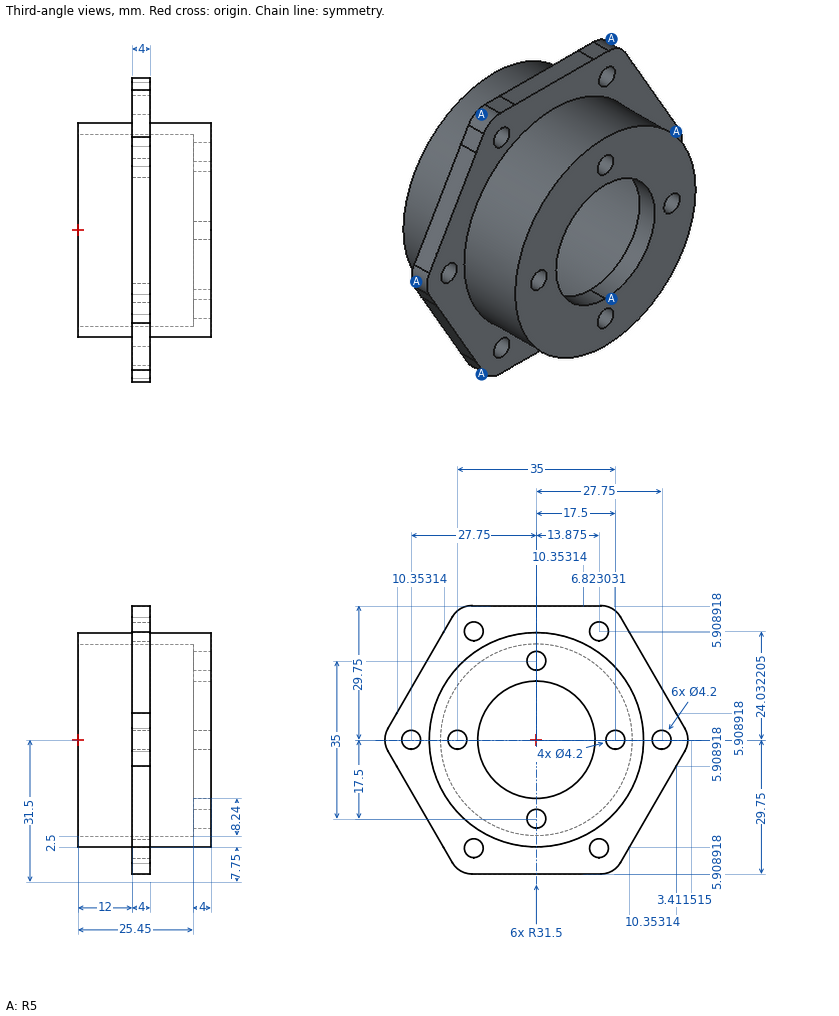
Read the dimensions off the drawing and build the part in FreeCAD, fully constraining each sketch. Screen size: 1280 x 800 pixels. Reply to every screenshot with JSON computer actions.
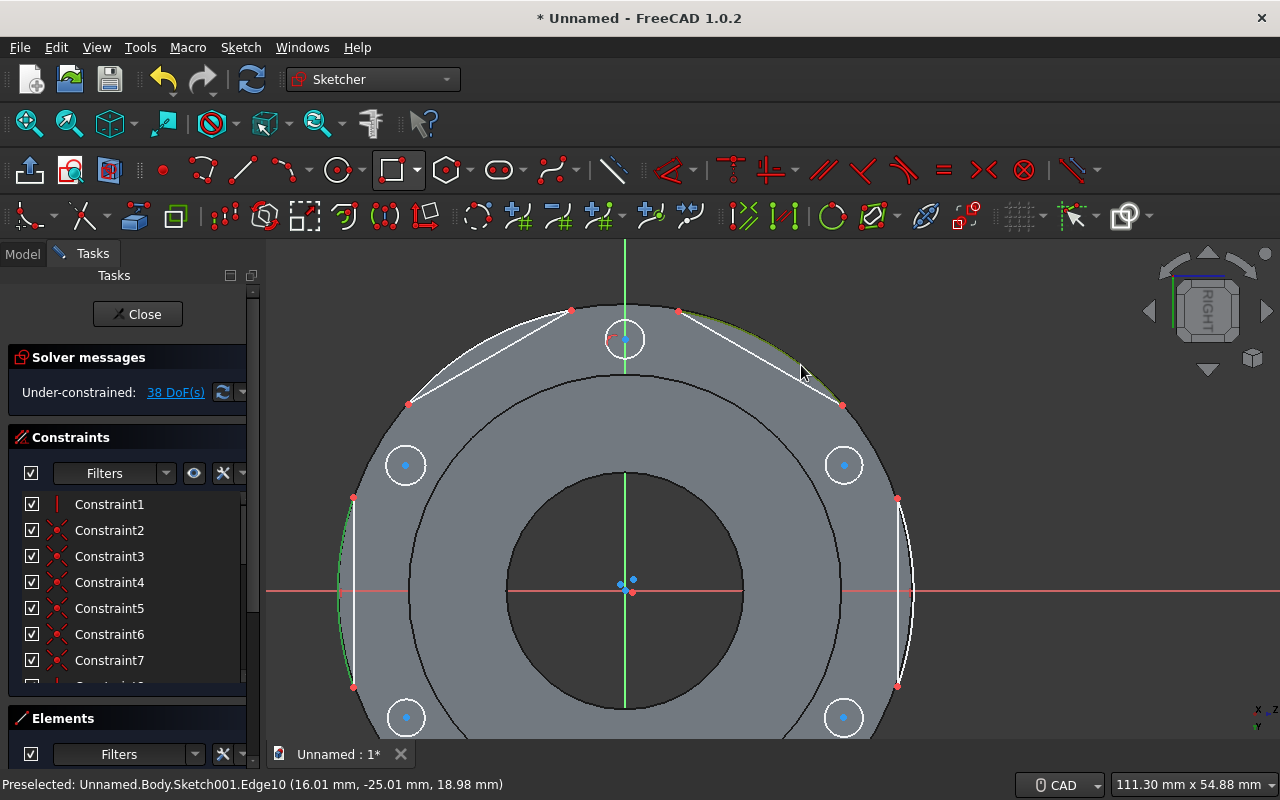
{"action": "key", "text": "c"}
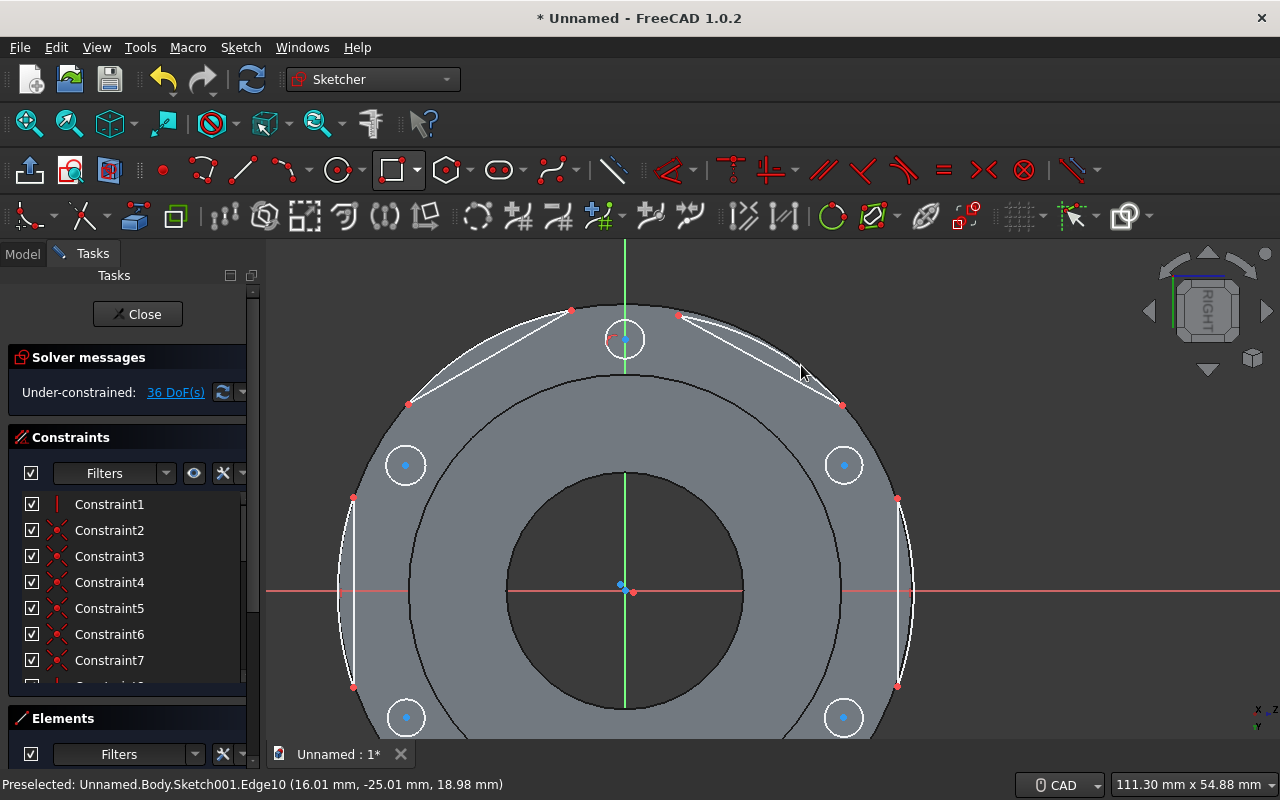
{"action": "left_click", "coordinate": [340, 554]}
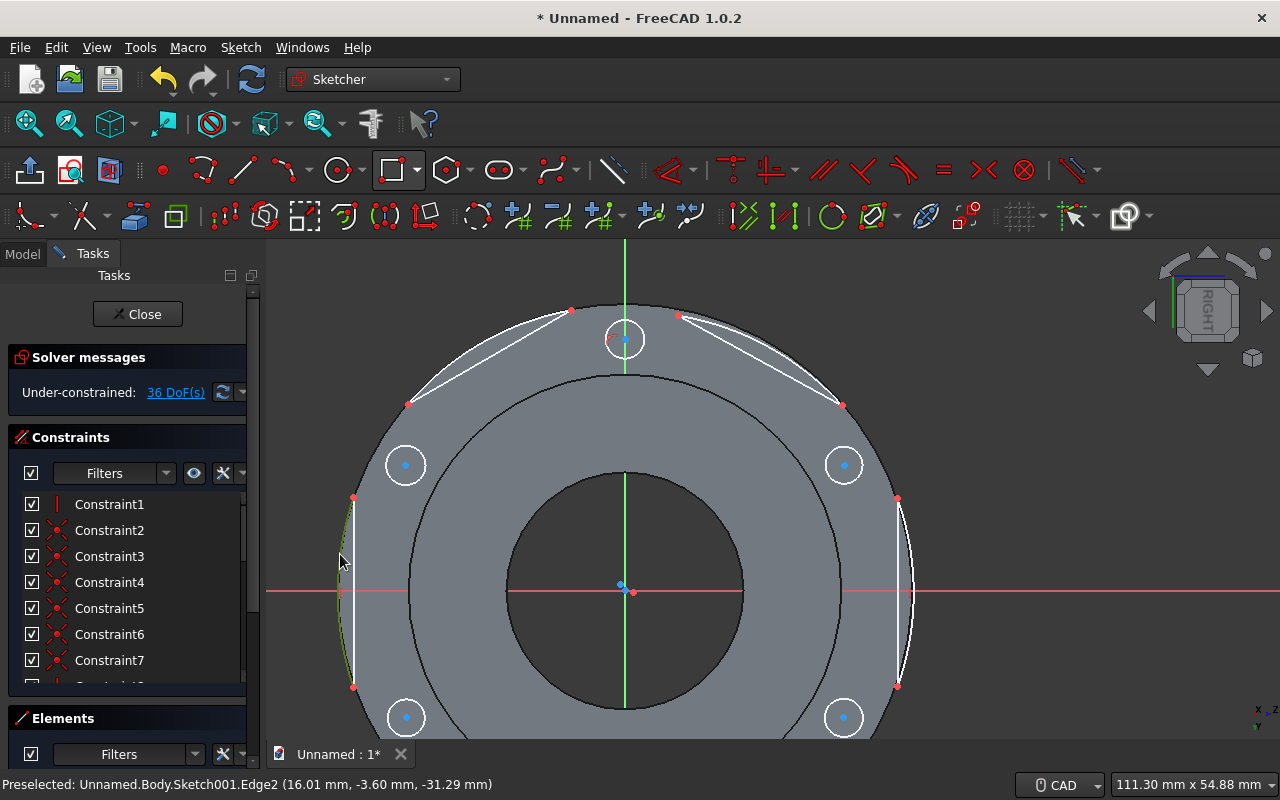
{"action": "left_click", "coordinate": [516, 326]}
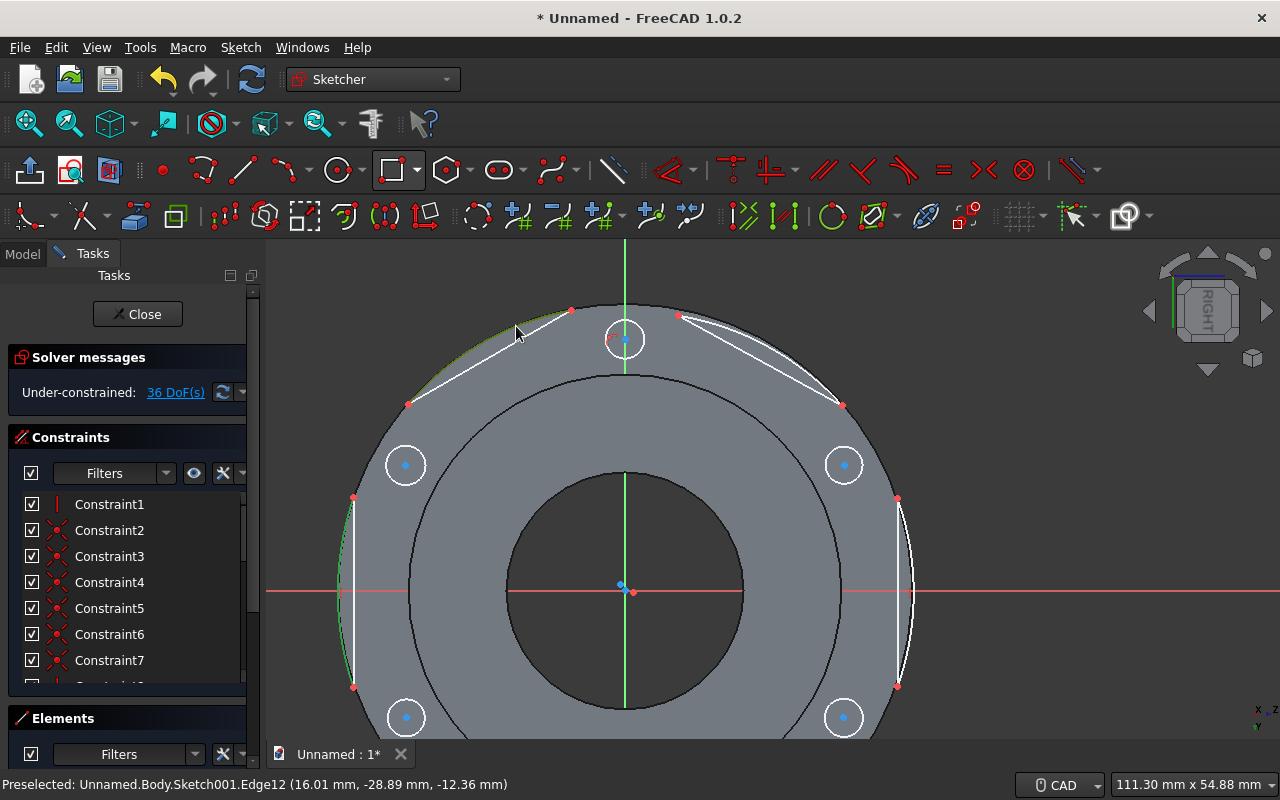
{"action": "key", "text": "c"}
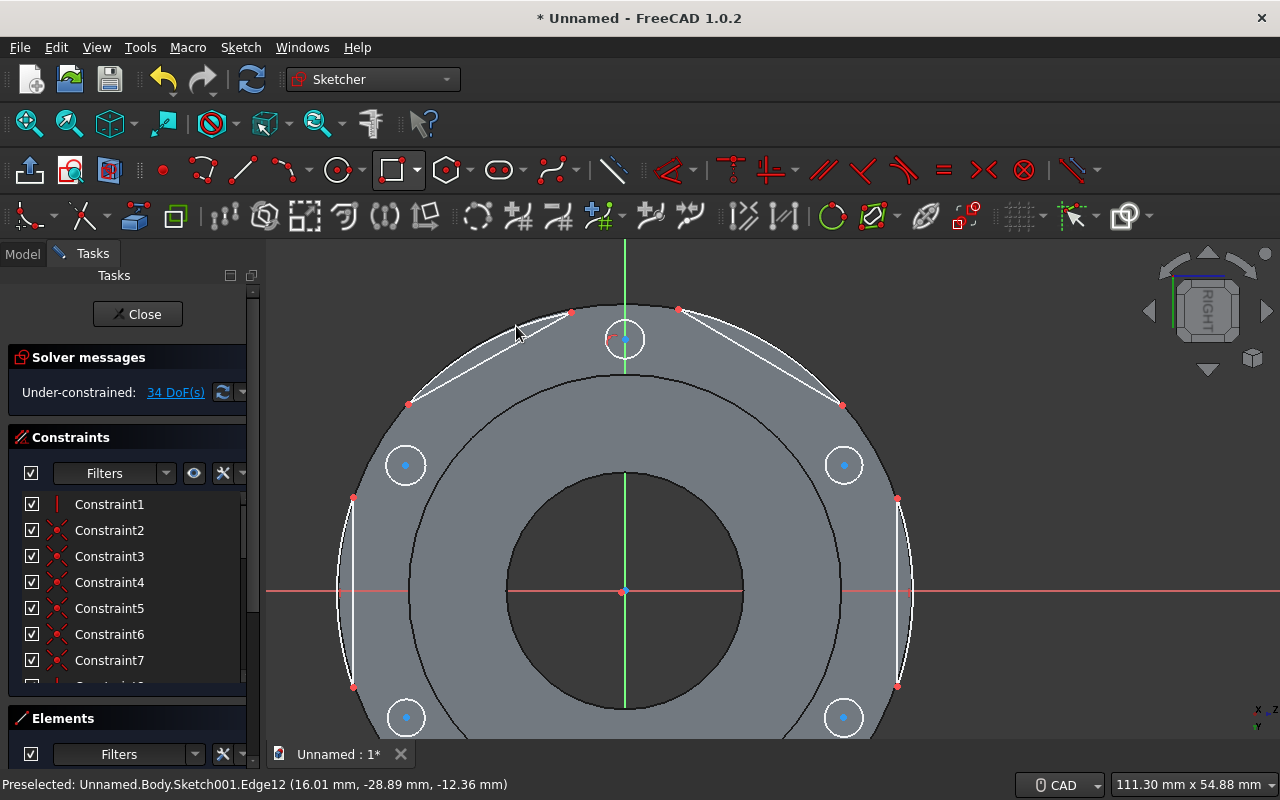
{"action": "scroll", "coordinate": [623, 592], "scroll_direction": "up", "scroll_amount": 4}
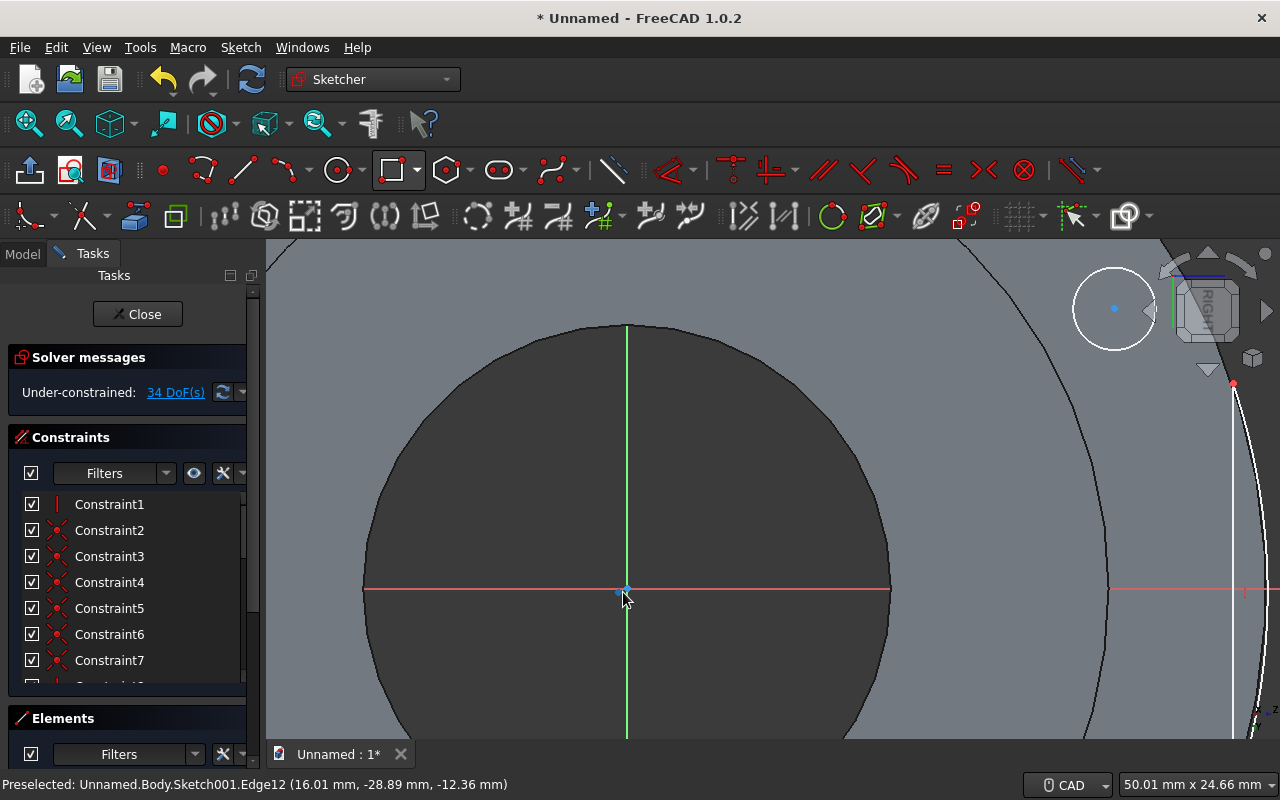
{"action": "left_click_drag", "start_coordinate": [609, 579], "coordinate": [637, 603]}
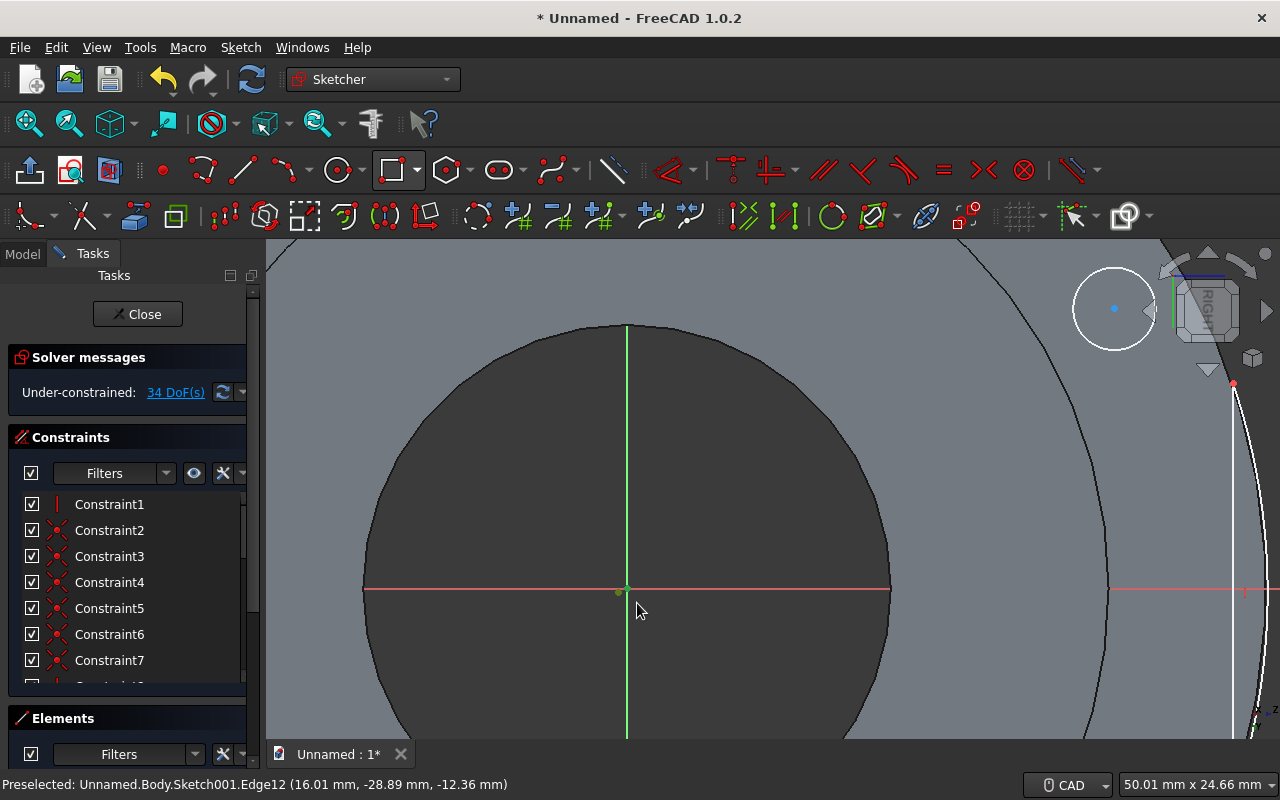
{"action": "key", "text": "c"}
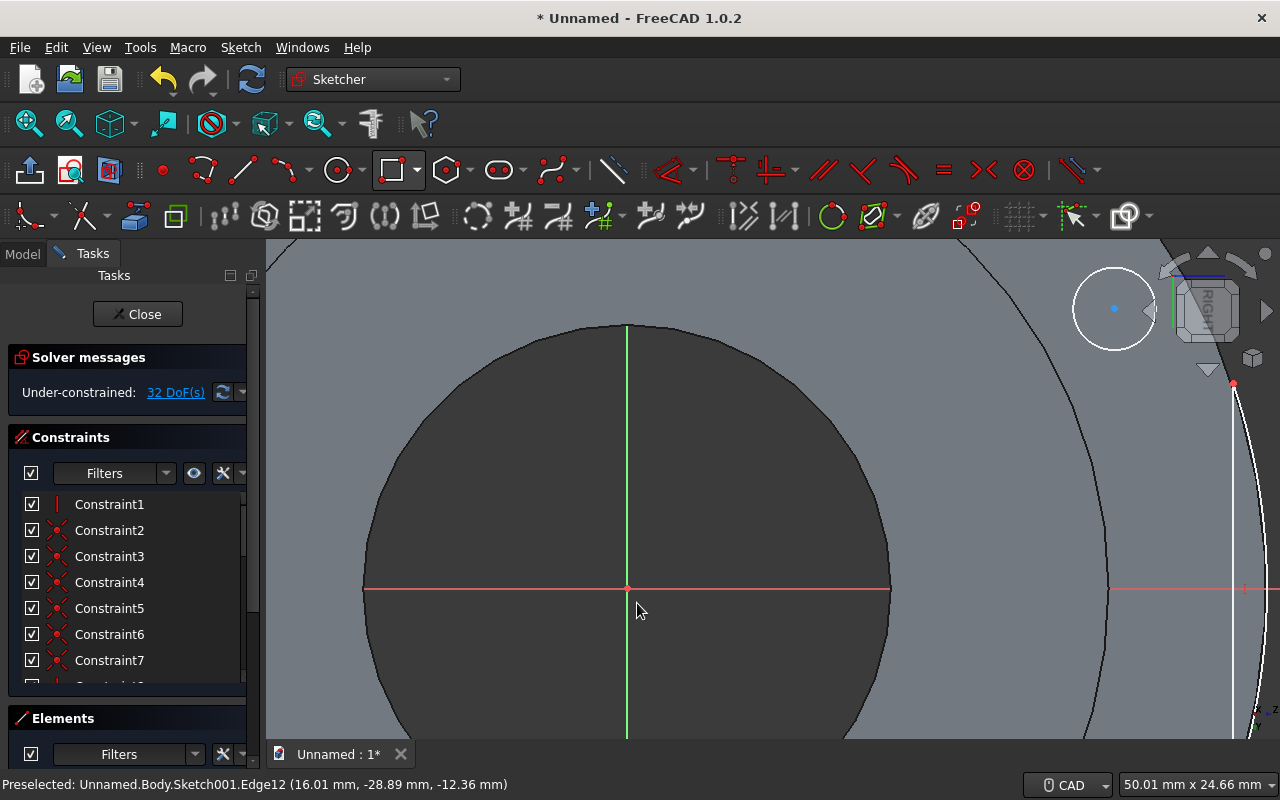
{"action": "scroll", "coordinate": [730, 456], "scroll_direction": "down", "scroll_amount": 7}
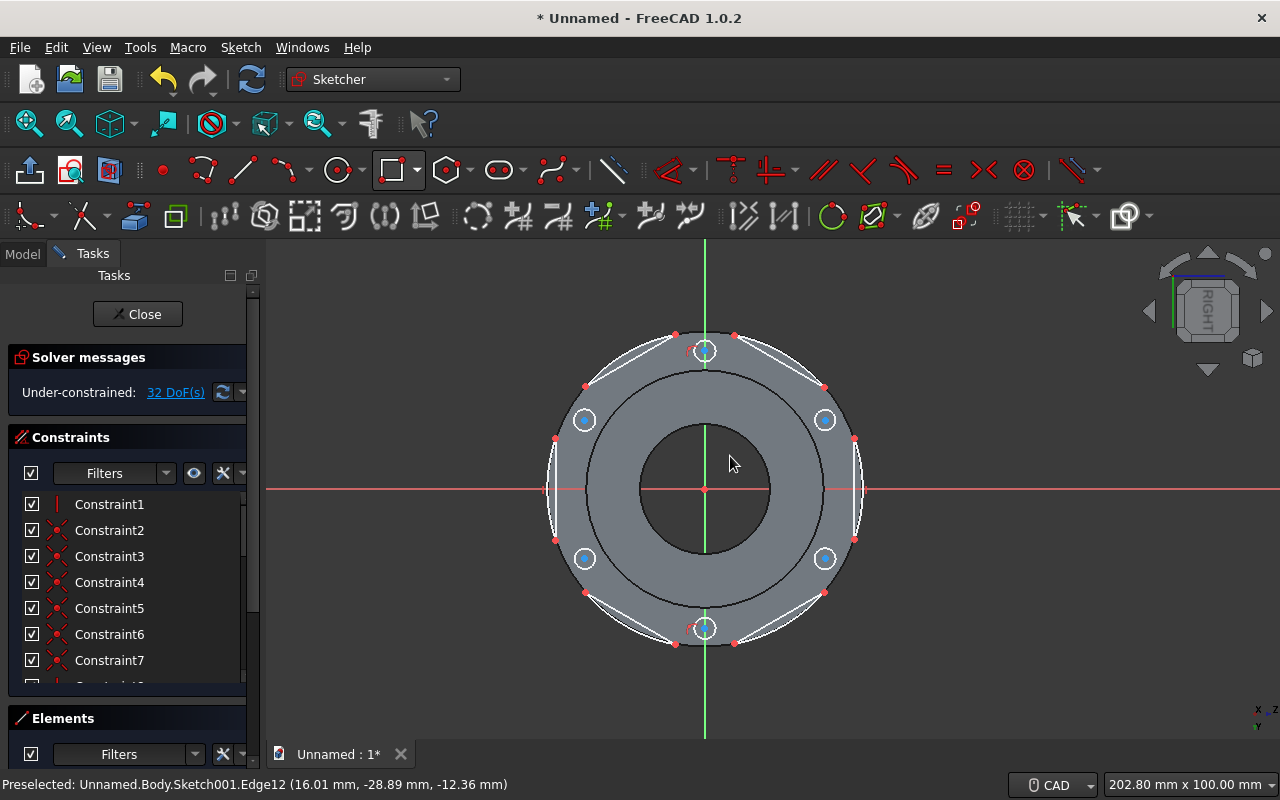
{"action": "scroll", "coordinate": [549, 468], "scroll_direction": "up", "scroll_amount": 4}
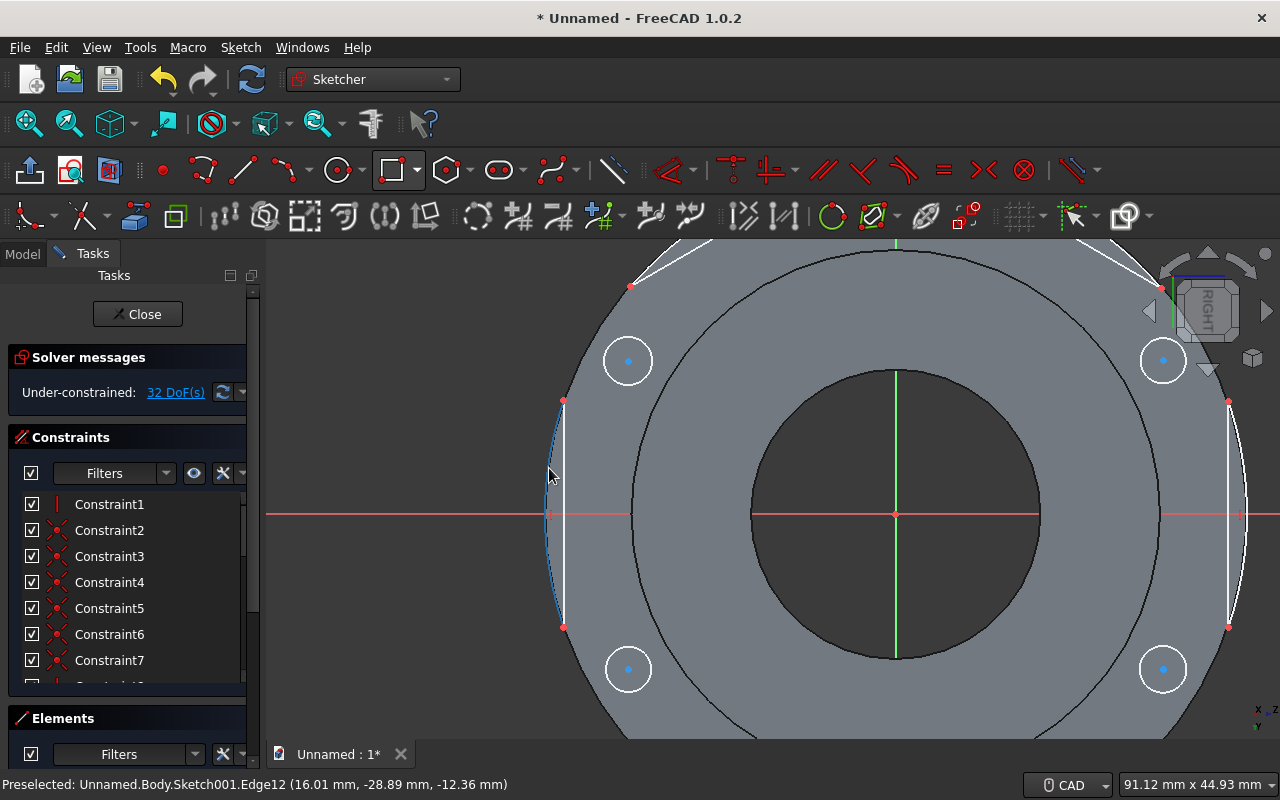
{"action": "left_click", "coordinate": [548, 468]}